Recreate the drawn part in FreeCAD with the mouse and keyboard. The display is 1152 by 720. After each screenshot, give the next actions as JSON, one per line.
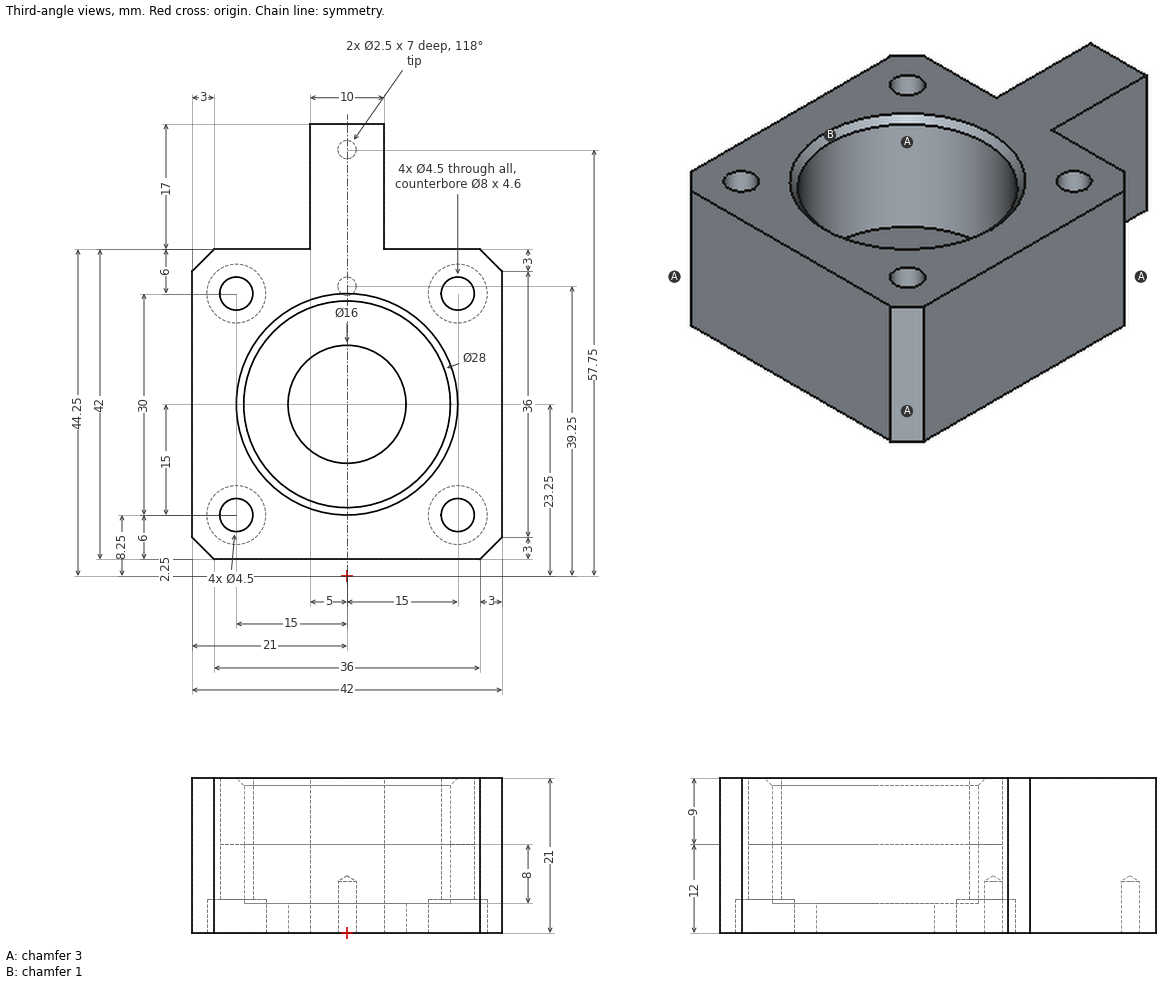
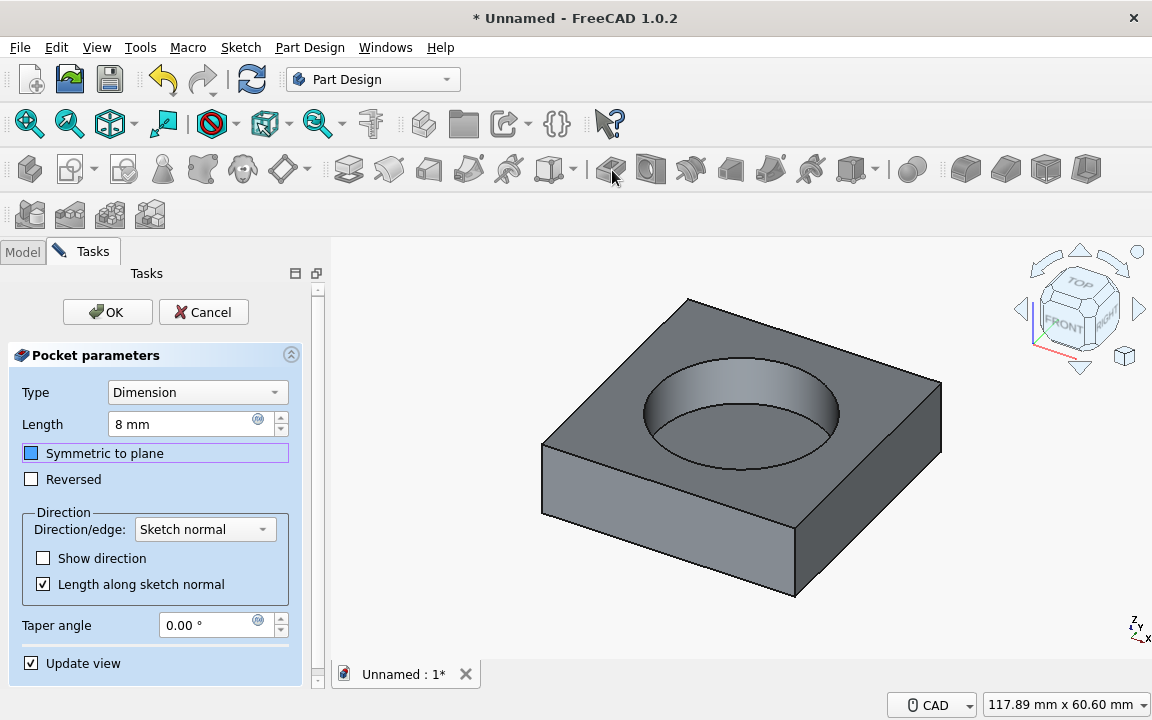
{"action": "left_click", "coordinate": [108, 312]}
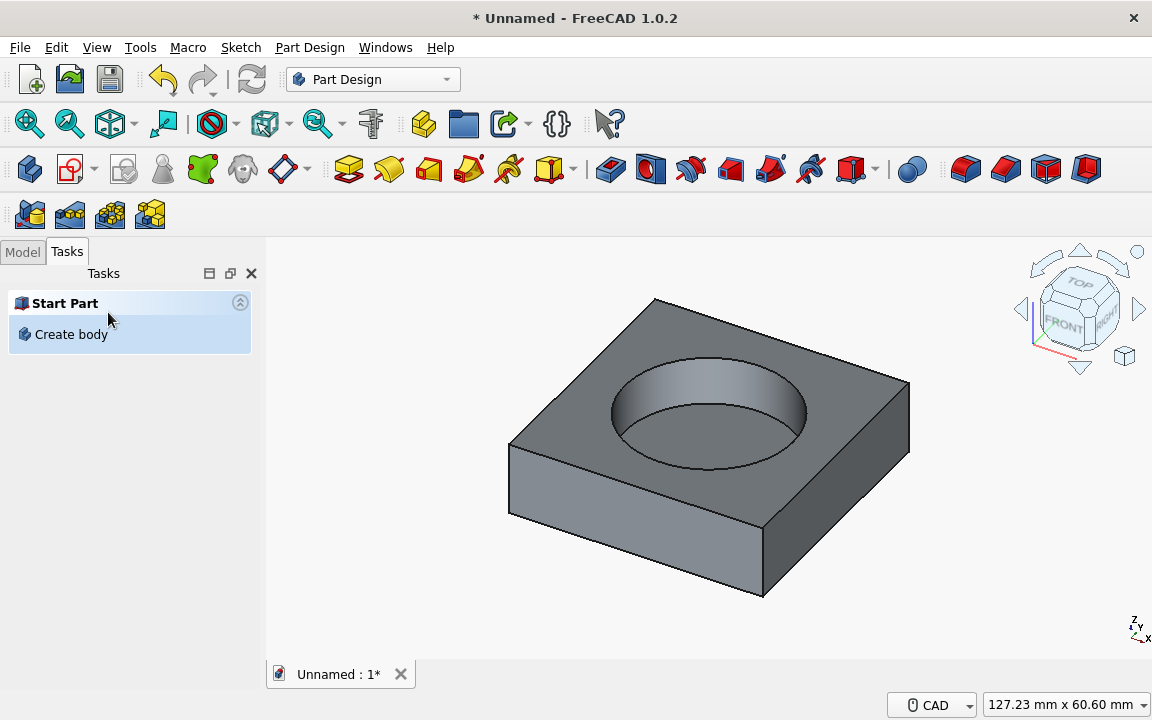
{"action": "left_click", "coordinate": [709, 458]}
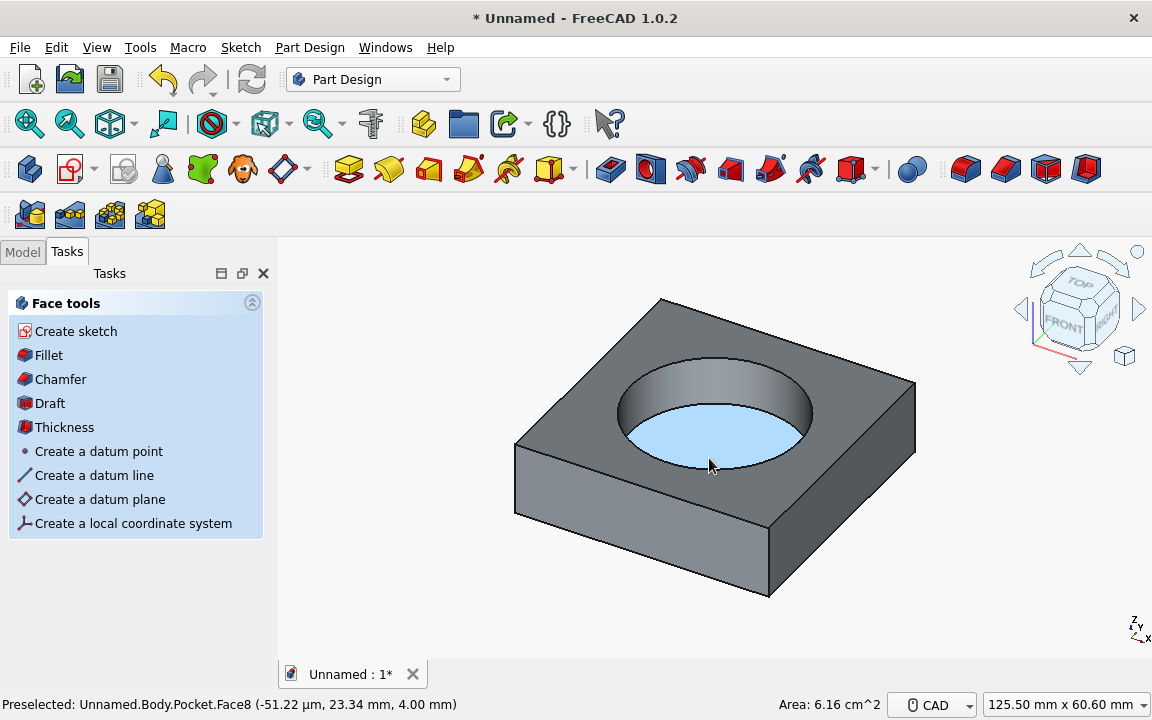
{"action": "left_click", "coordinate": [70, 170]}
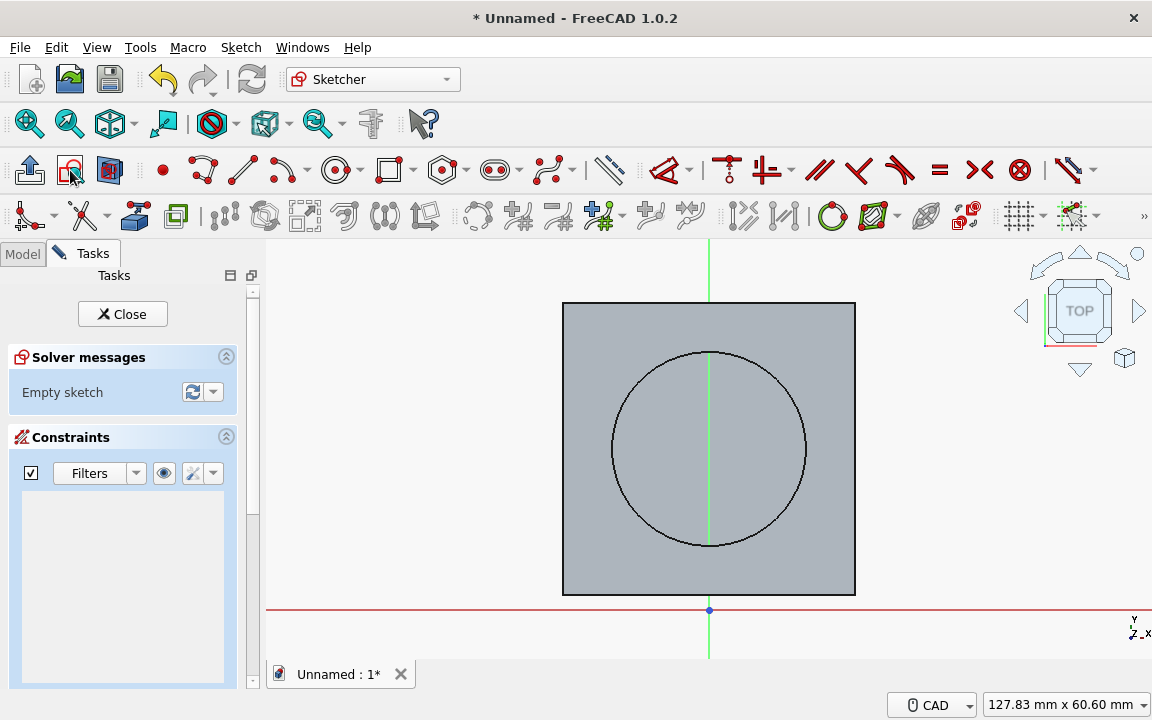
{"action": "scroll", "coordinate": [987, 631], "scroll_direction": "up", "scroll_amount": 1}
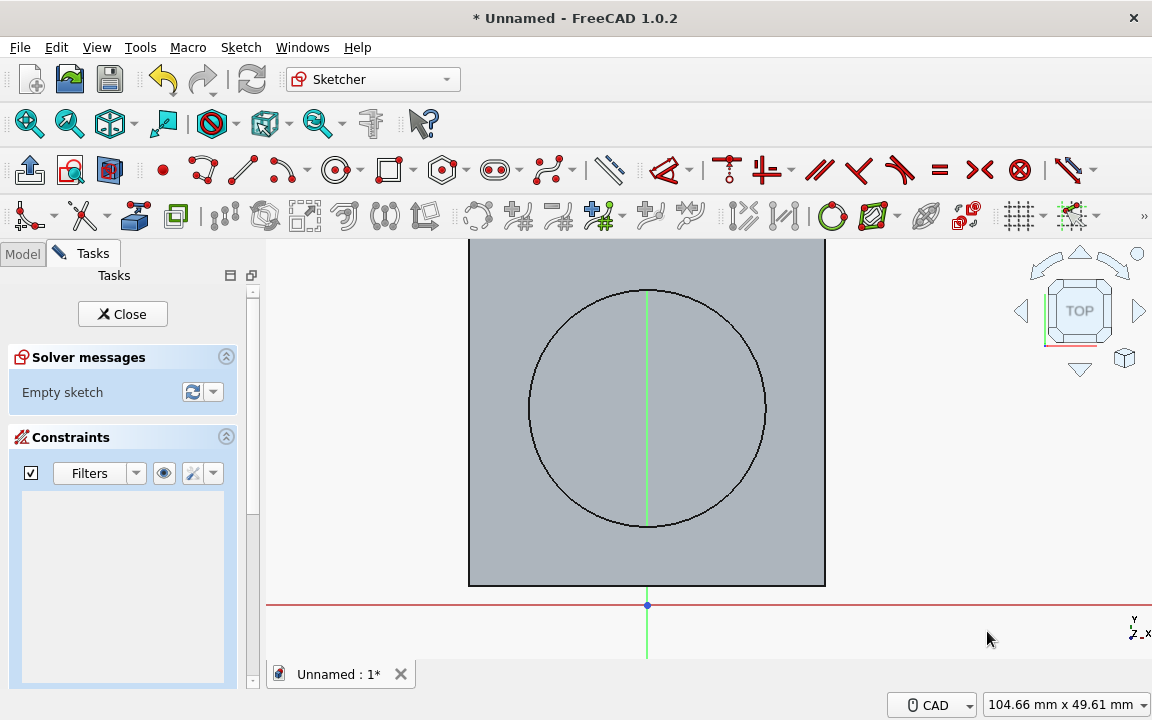
{"action": "left_click", "coordinate": [336, 170]}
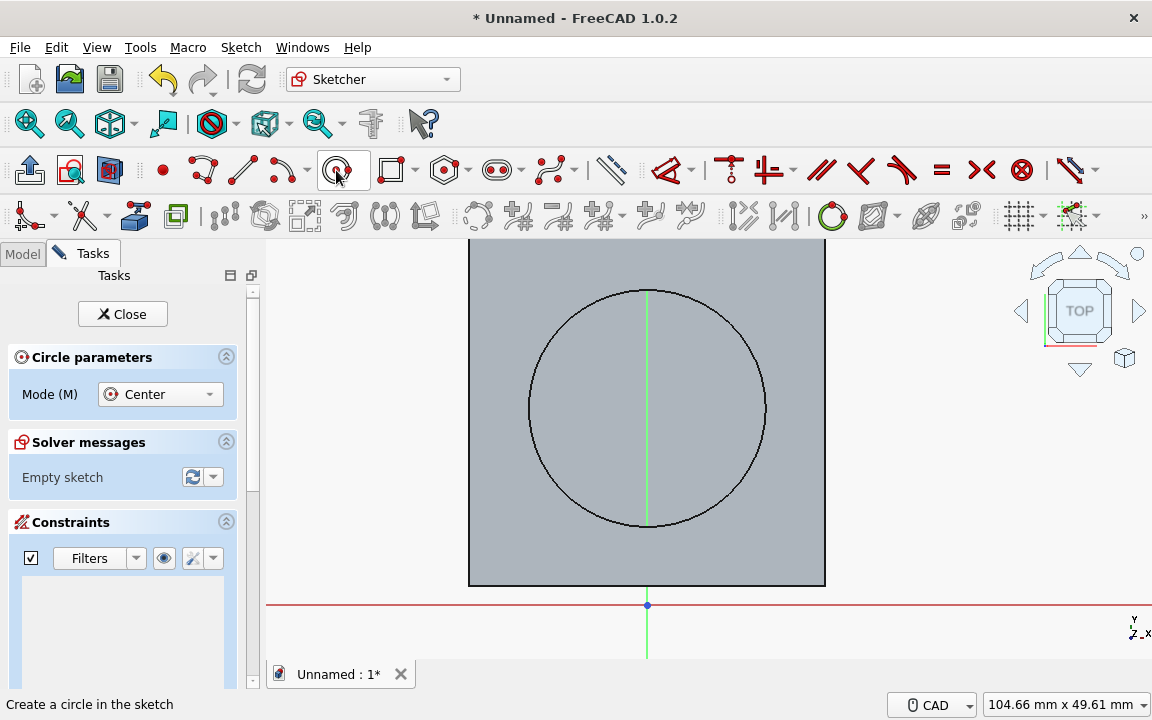
{"action": "left_click", "coordinate": [647, 408]}
{"action": "left_click", "coordinate": [695, 361]}
{"action": "key", "text": "Escape"}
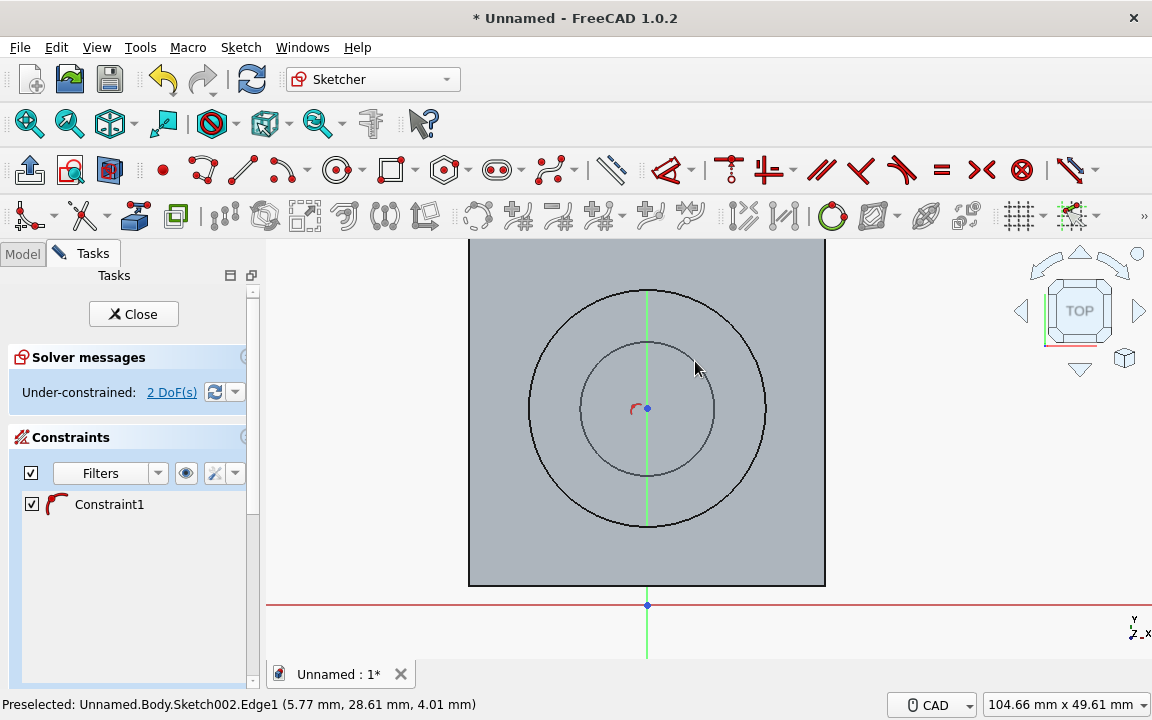
{"action": "left_click", "coordinate": [666, 170]}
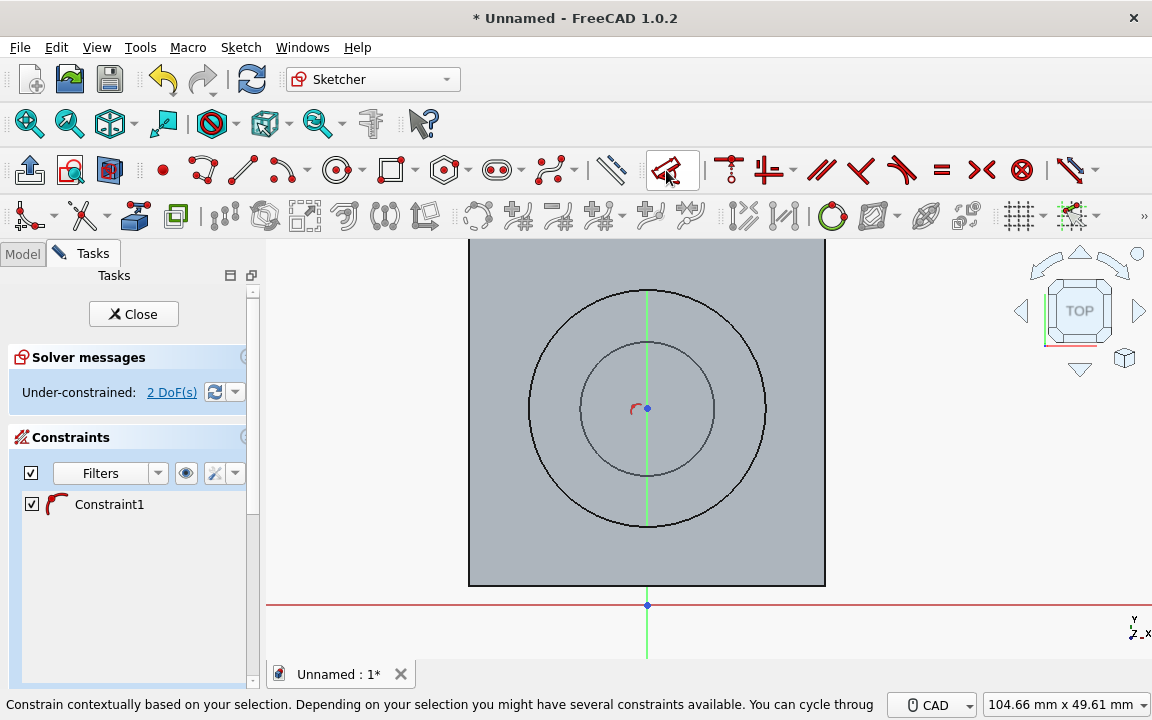
{"action": "left_click", "coordinate": [694, 361]}
{"action": "left_click", "coordinate": [716, 338]}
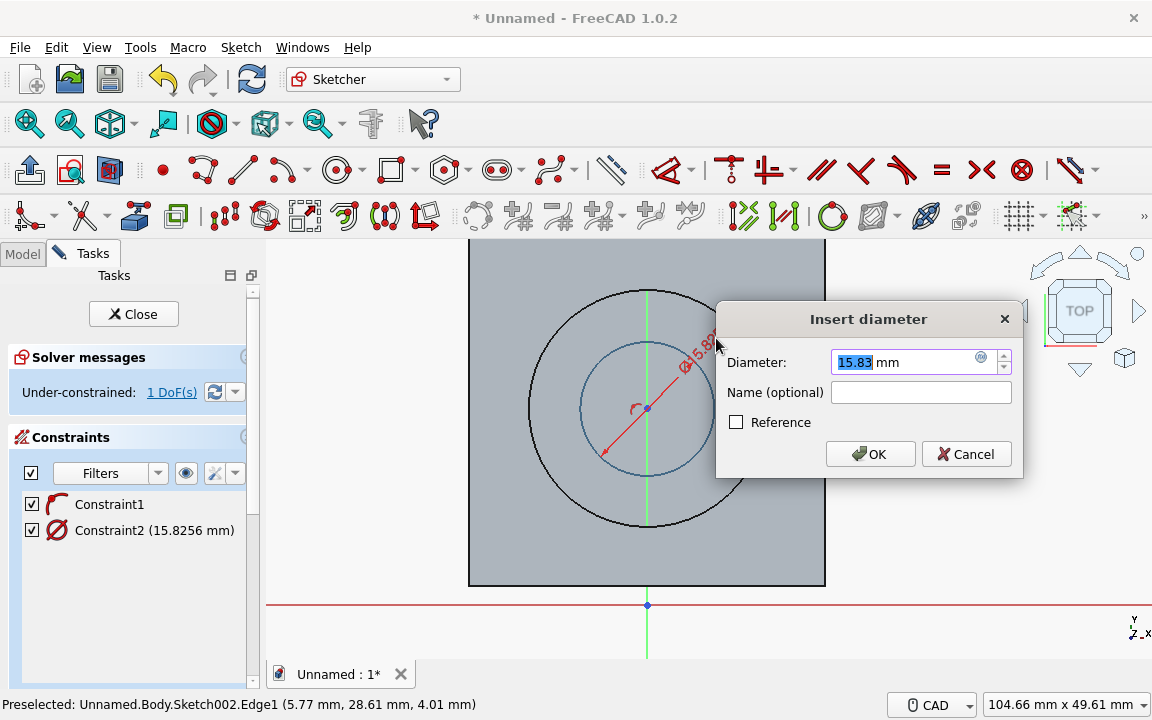
{"action": "type", "text": "16"}
{"action": "key", "text": "Return"}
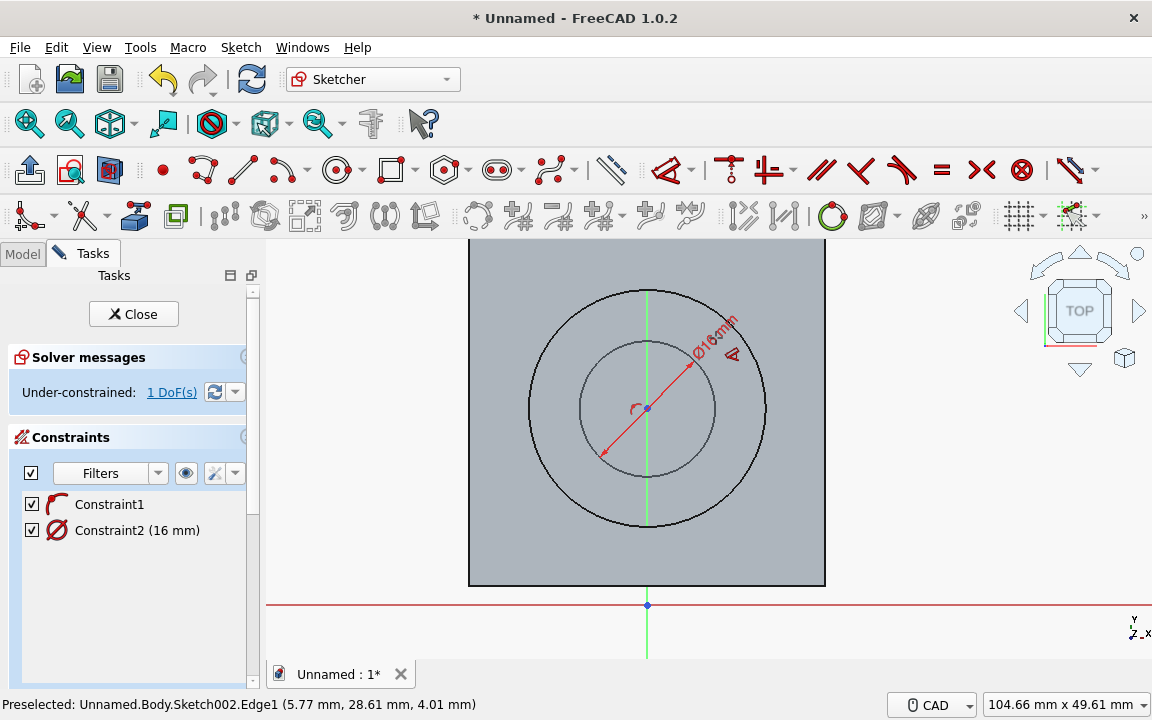
{"action": "left_click", "coordinate": [647, 409]}
{"action": "left_click", "coordinate": [681, 507]}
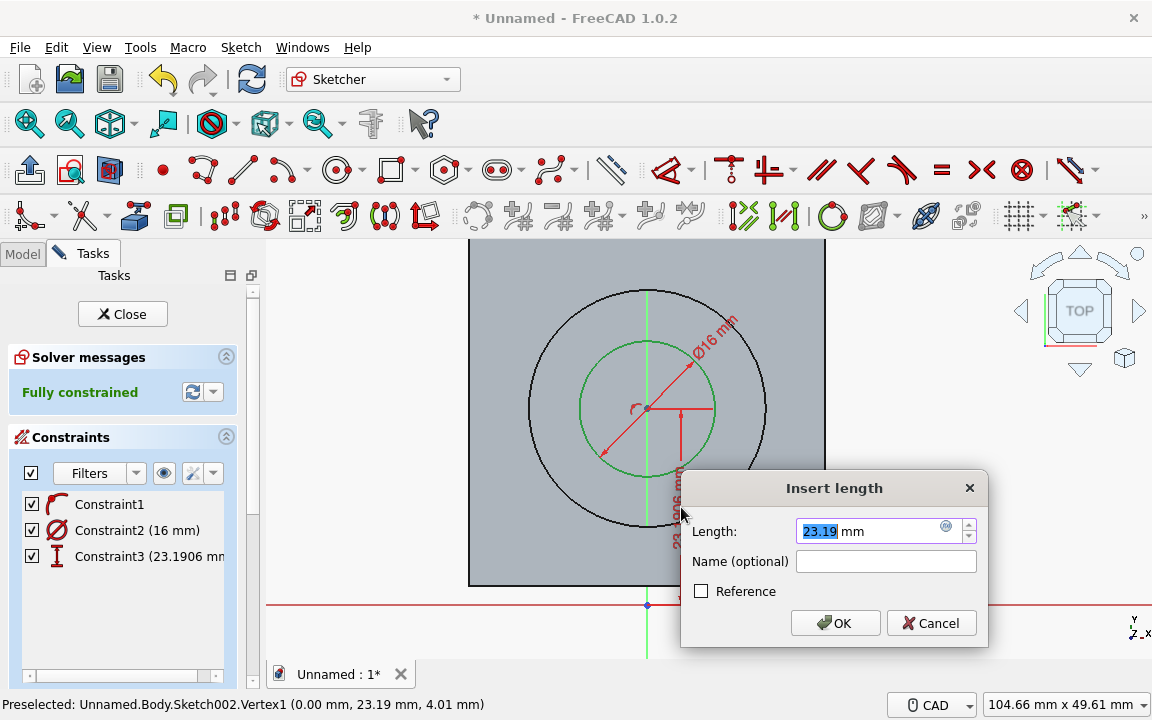
{"action": "type", "text": "23.25"}
{"action": "key", "text": "Return"}
{"action": "key", "text": "Escape"}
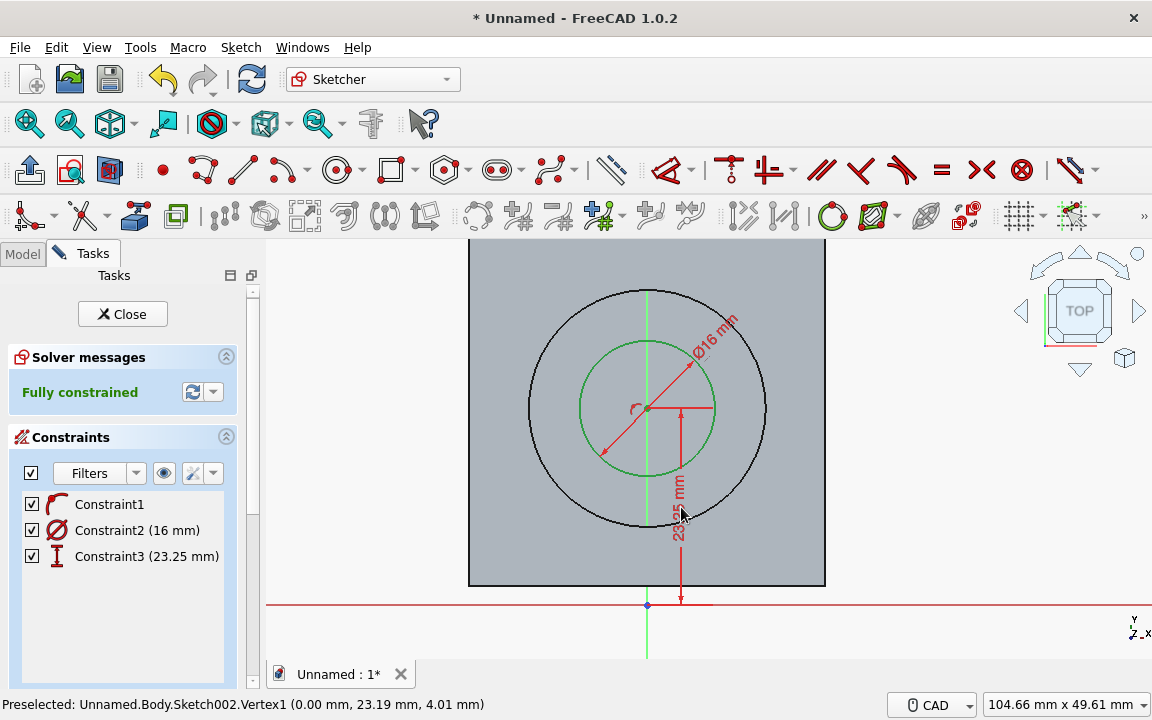
{"action": "left_click", "coordinate": [123, 314]}